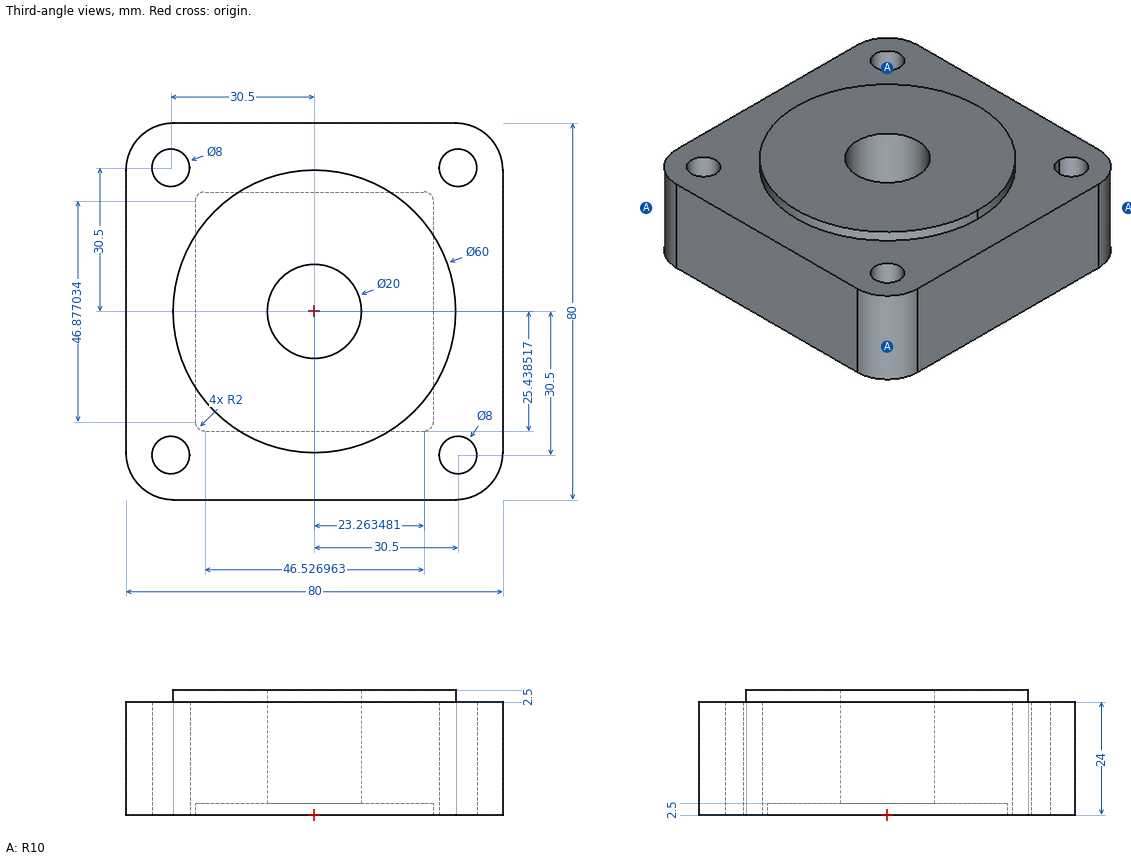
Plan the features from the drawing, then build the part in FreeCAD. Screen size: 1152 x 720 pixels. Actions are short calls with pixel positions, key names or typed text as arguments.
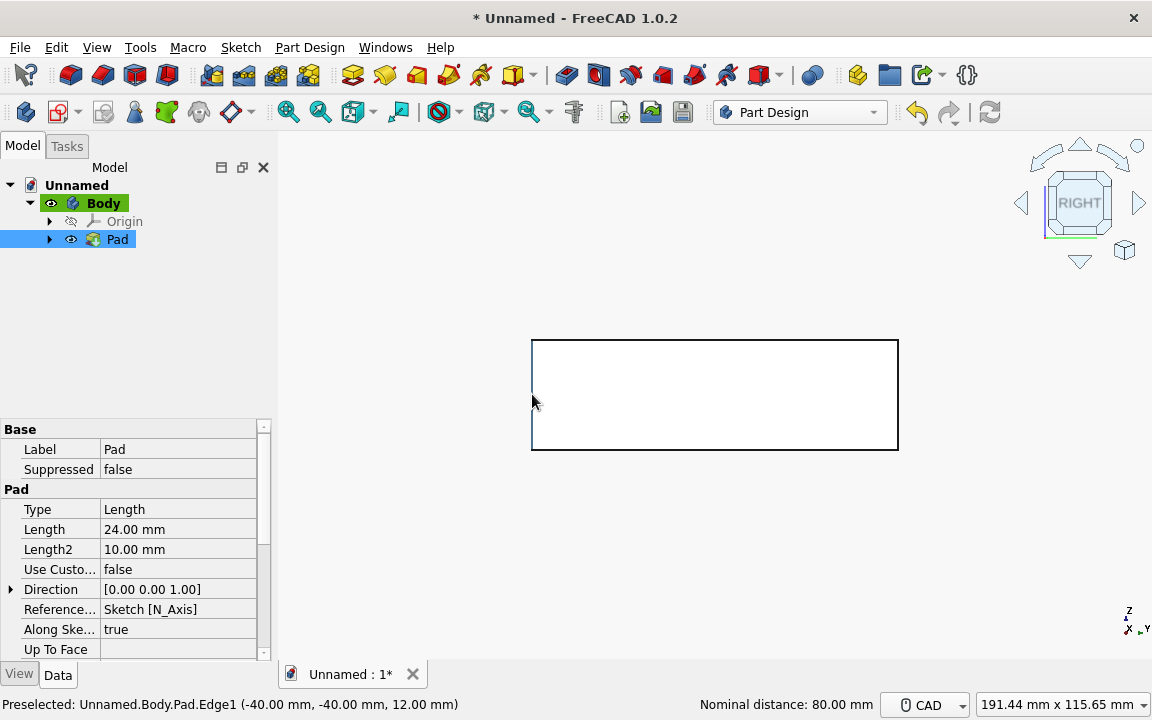
click(290, 112)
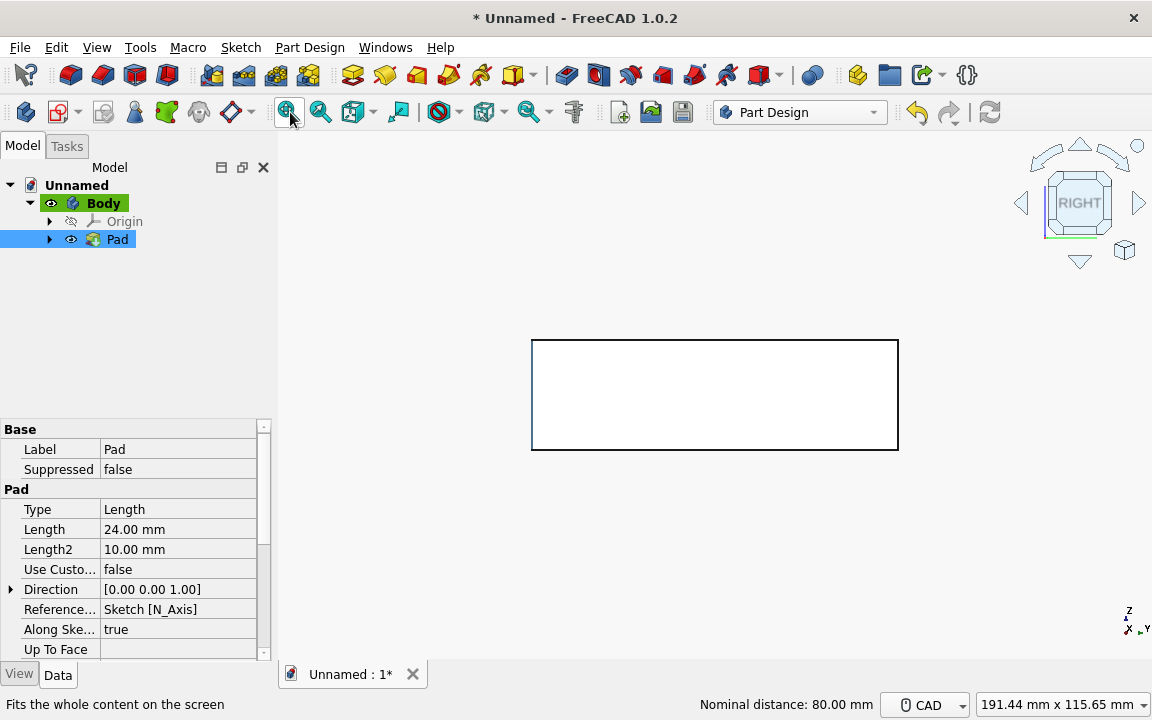
click(898, 394, ctrl)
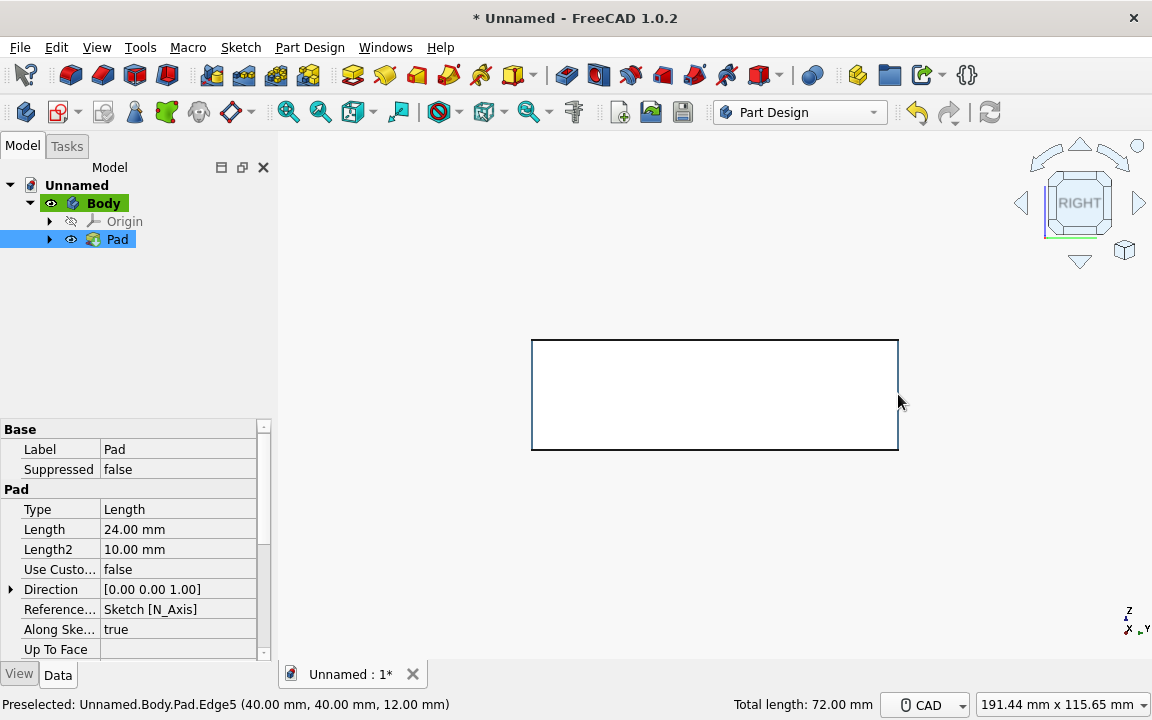
key(5)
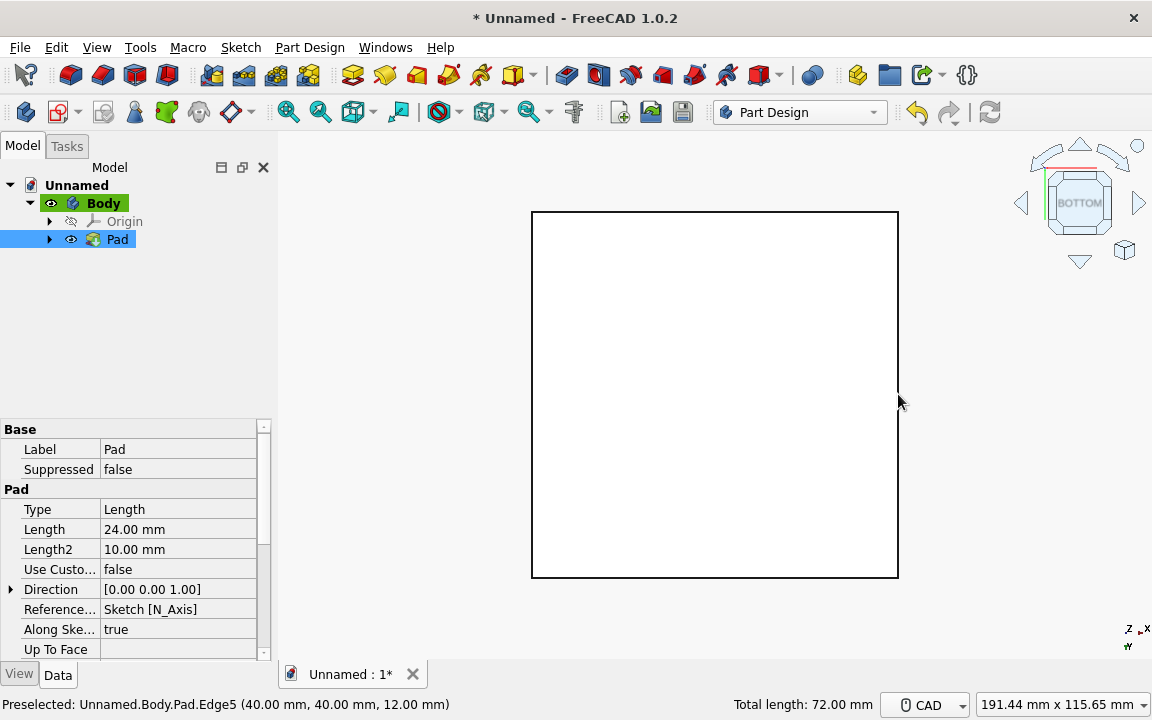
key(4)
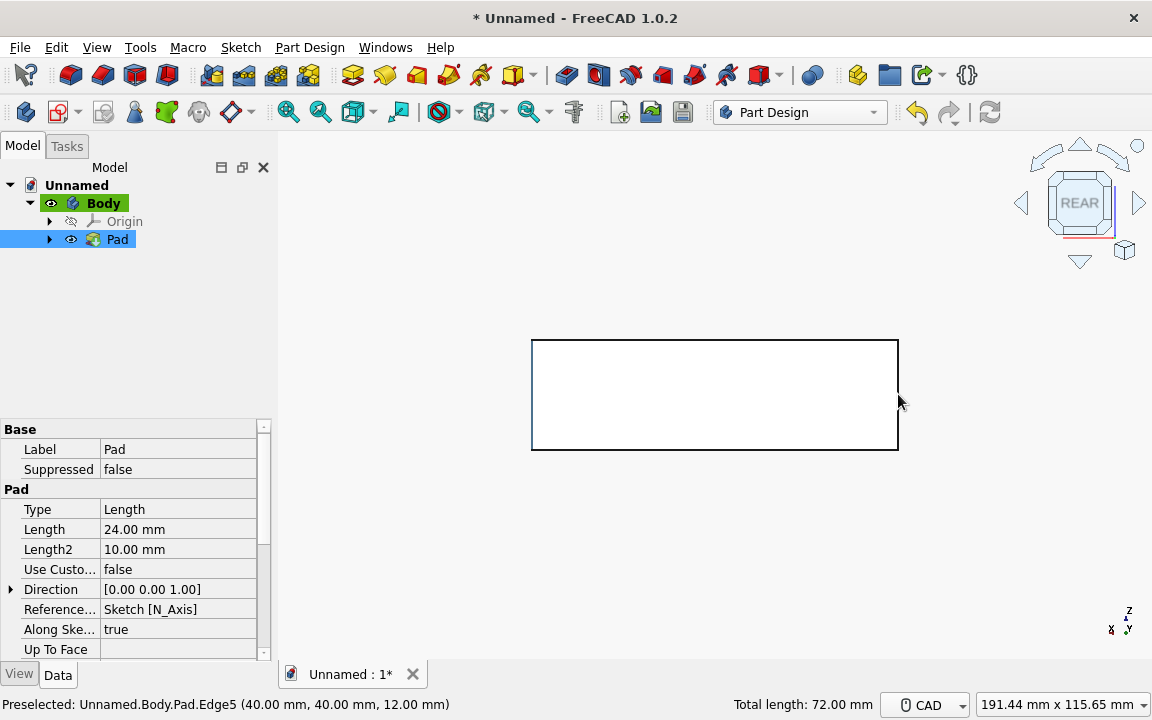
click(290, 112)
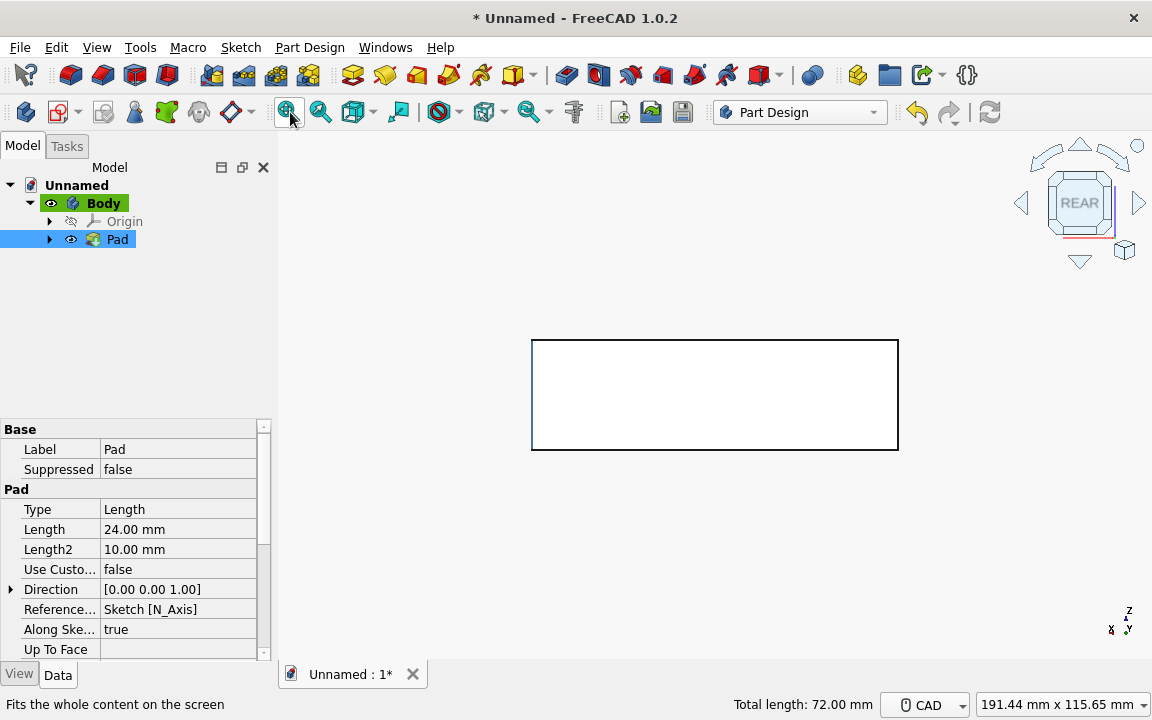
click(898, 394, ctrl)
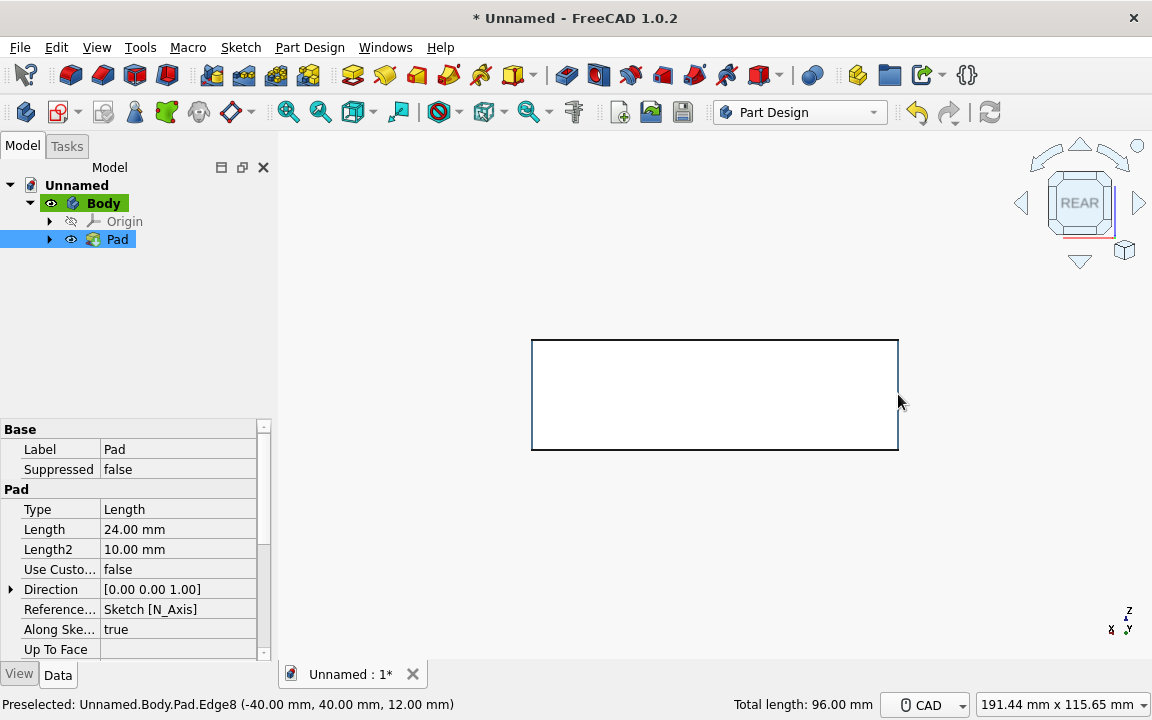
click(72, 76)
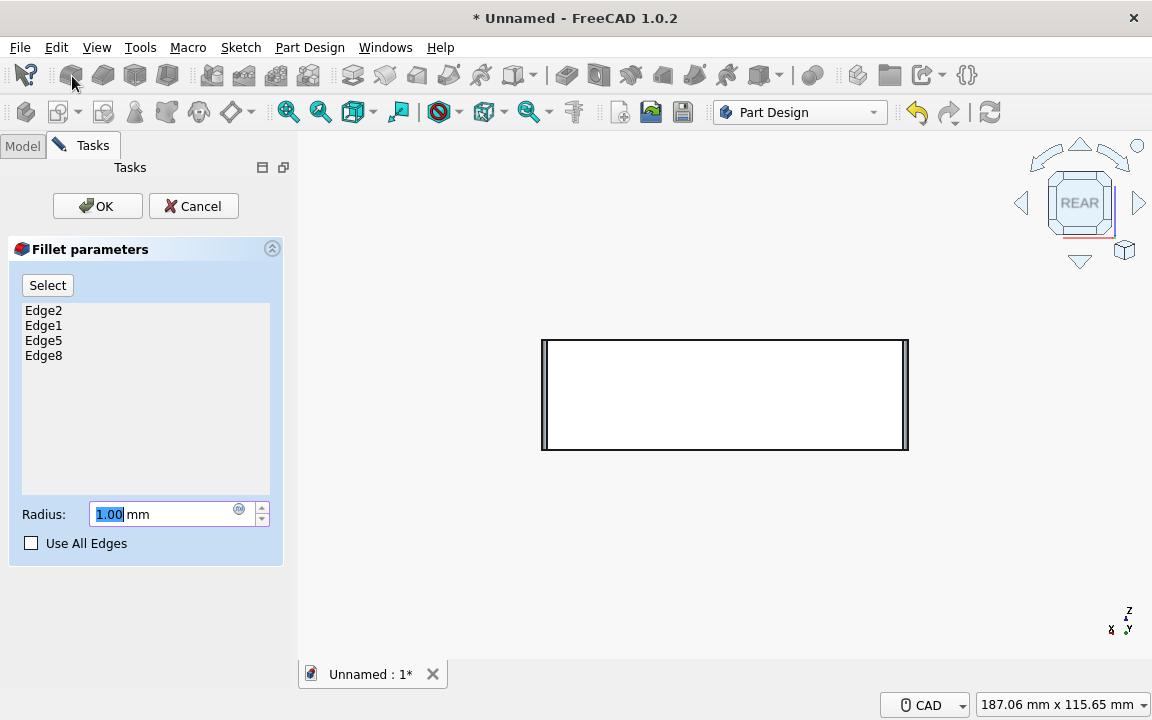
text(10)
key(Tab)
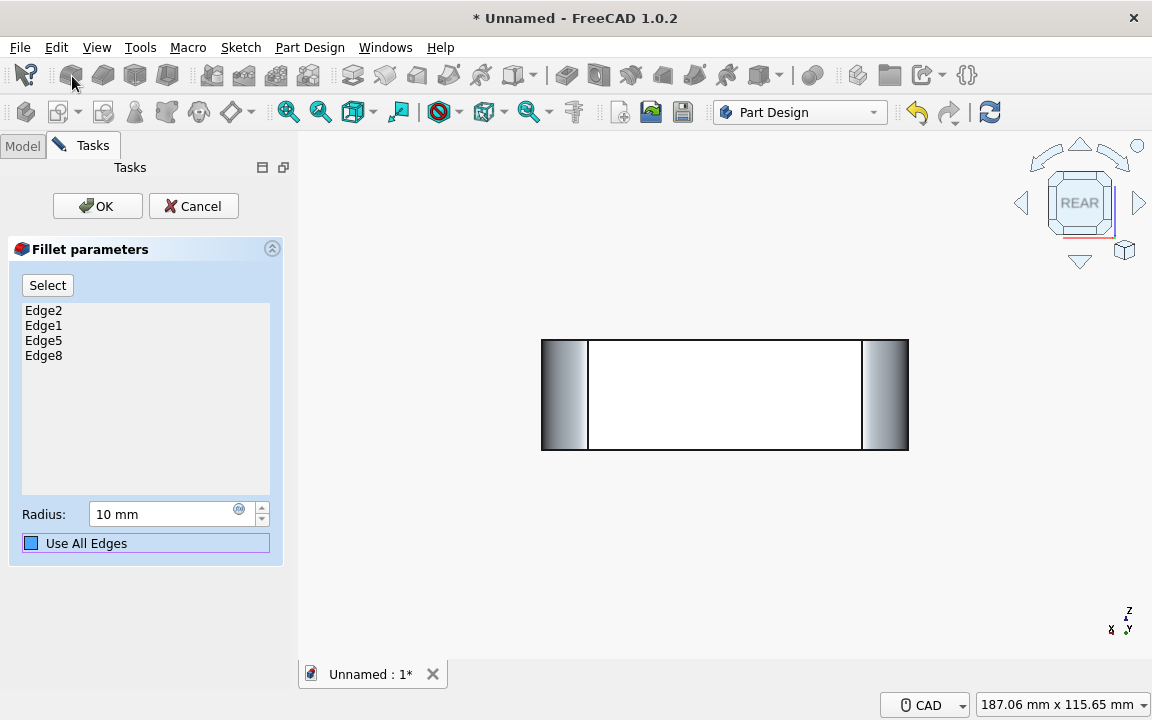
click(98, 206)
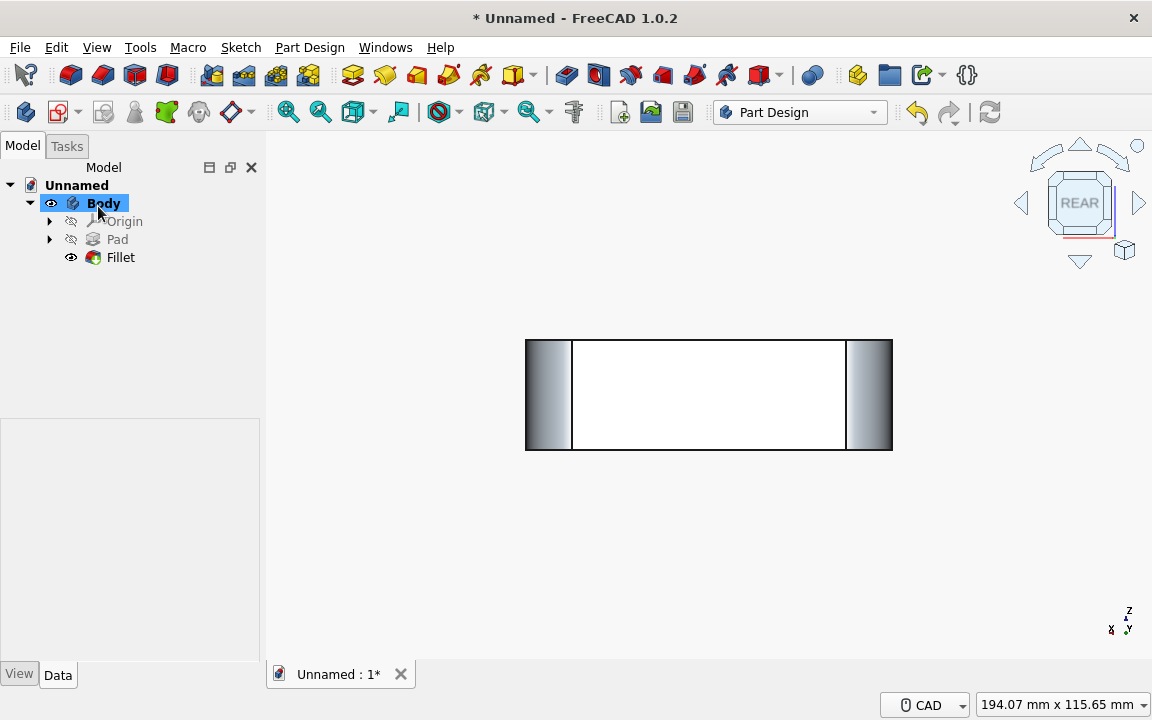
click(290, 112)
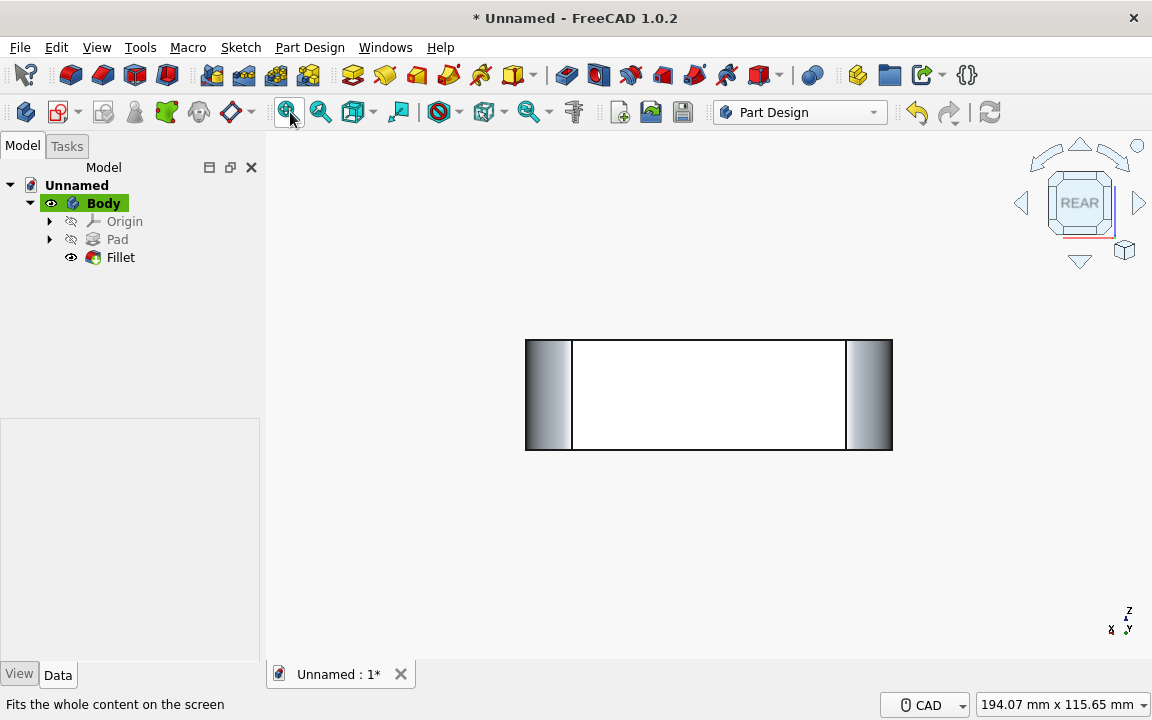
key(0)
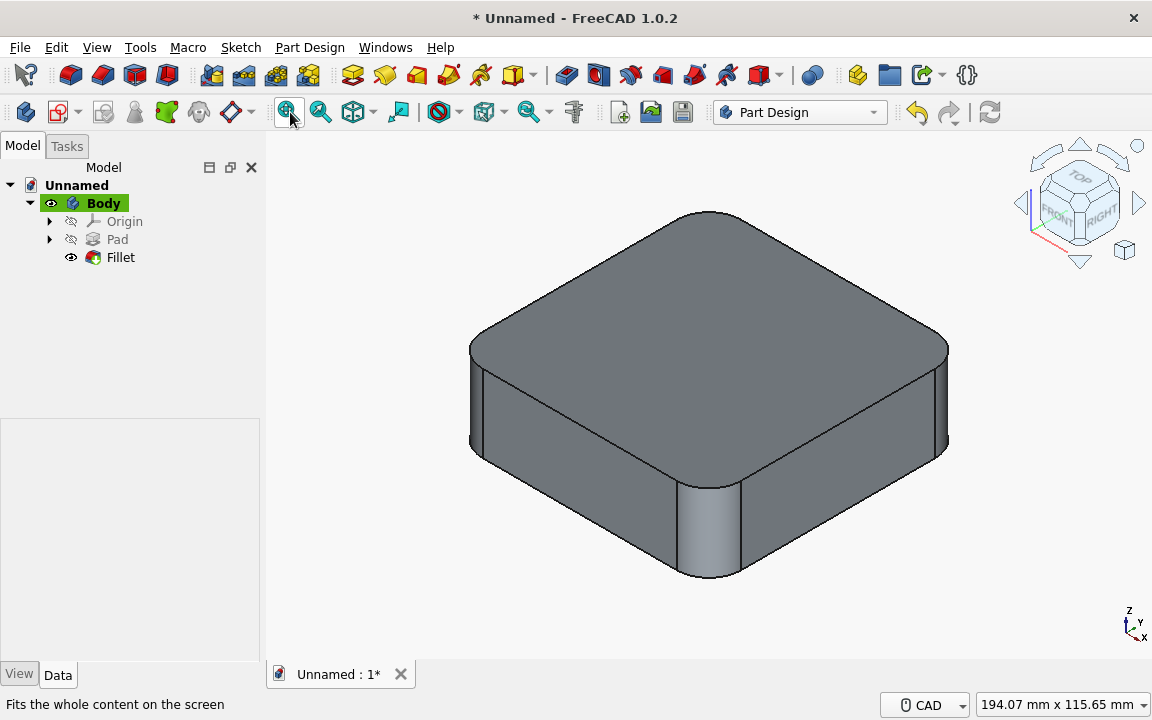
click(709, 349)